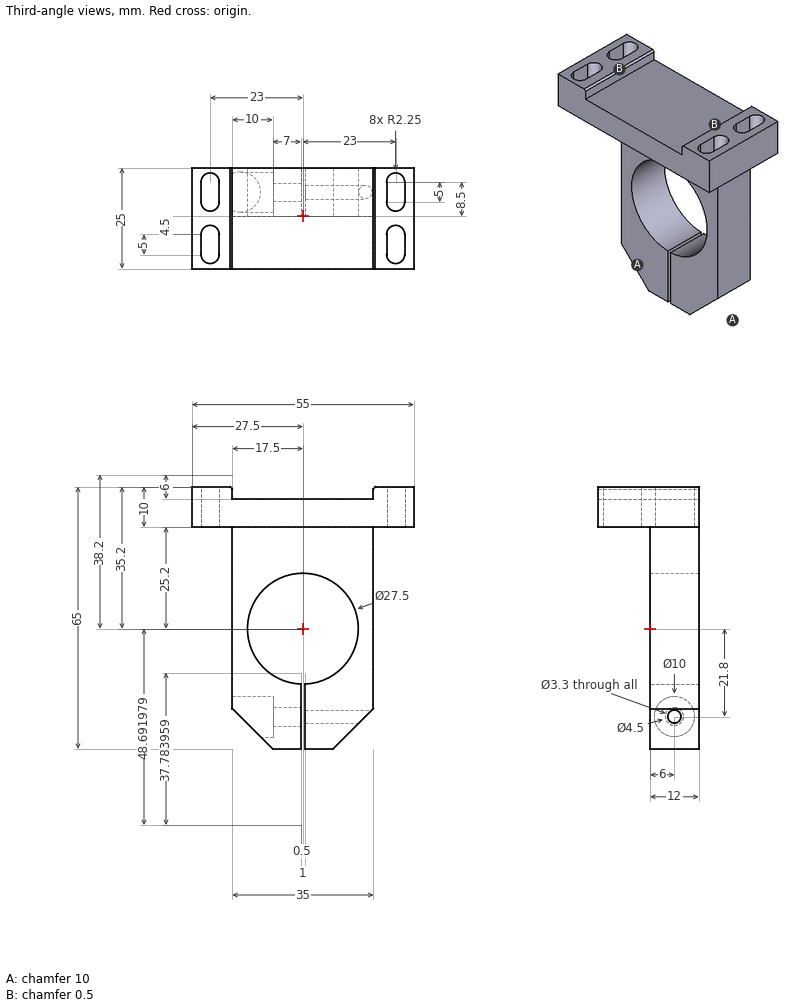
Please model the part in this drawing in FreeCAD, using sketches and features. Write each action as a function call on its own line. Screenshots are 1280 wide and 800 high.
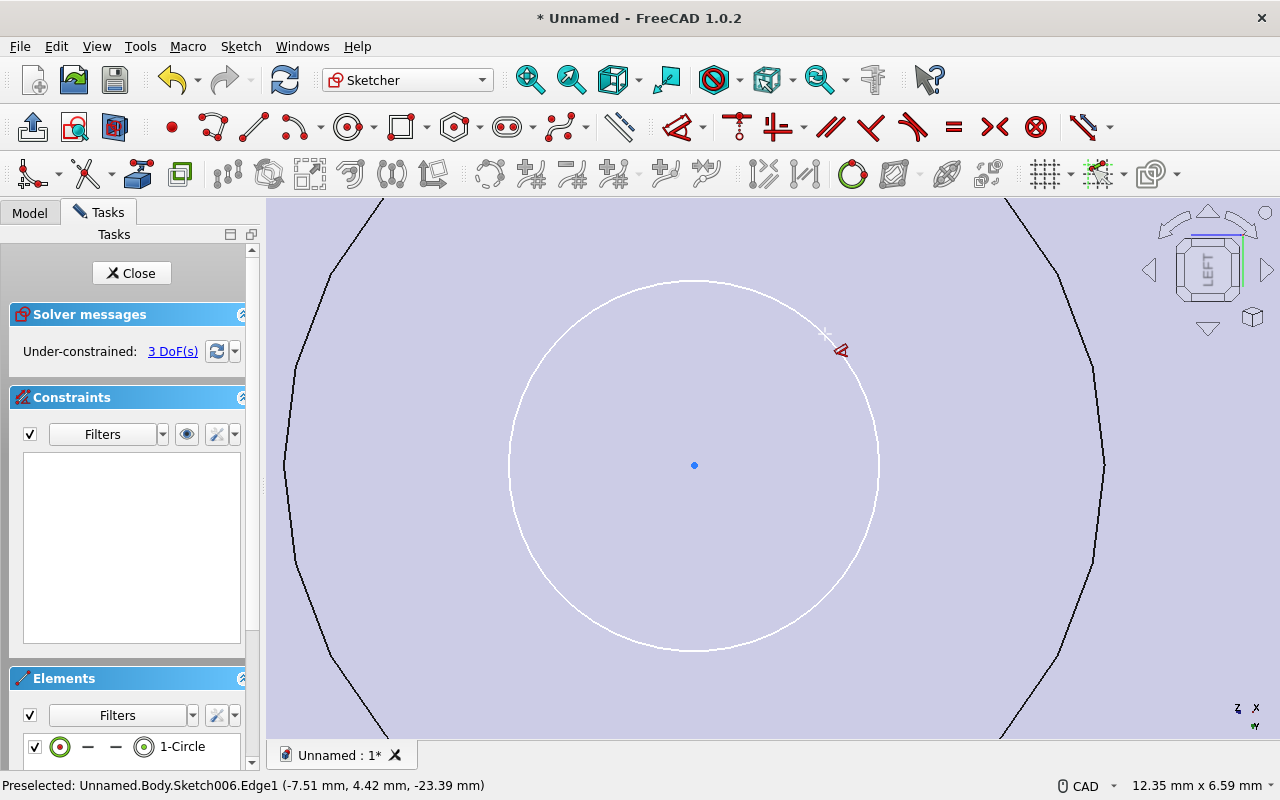
click(825, 335)
click(848, 312)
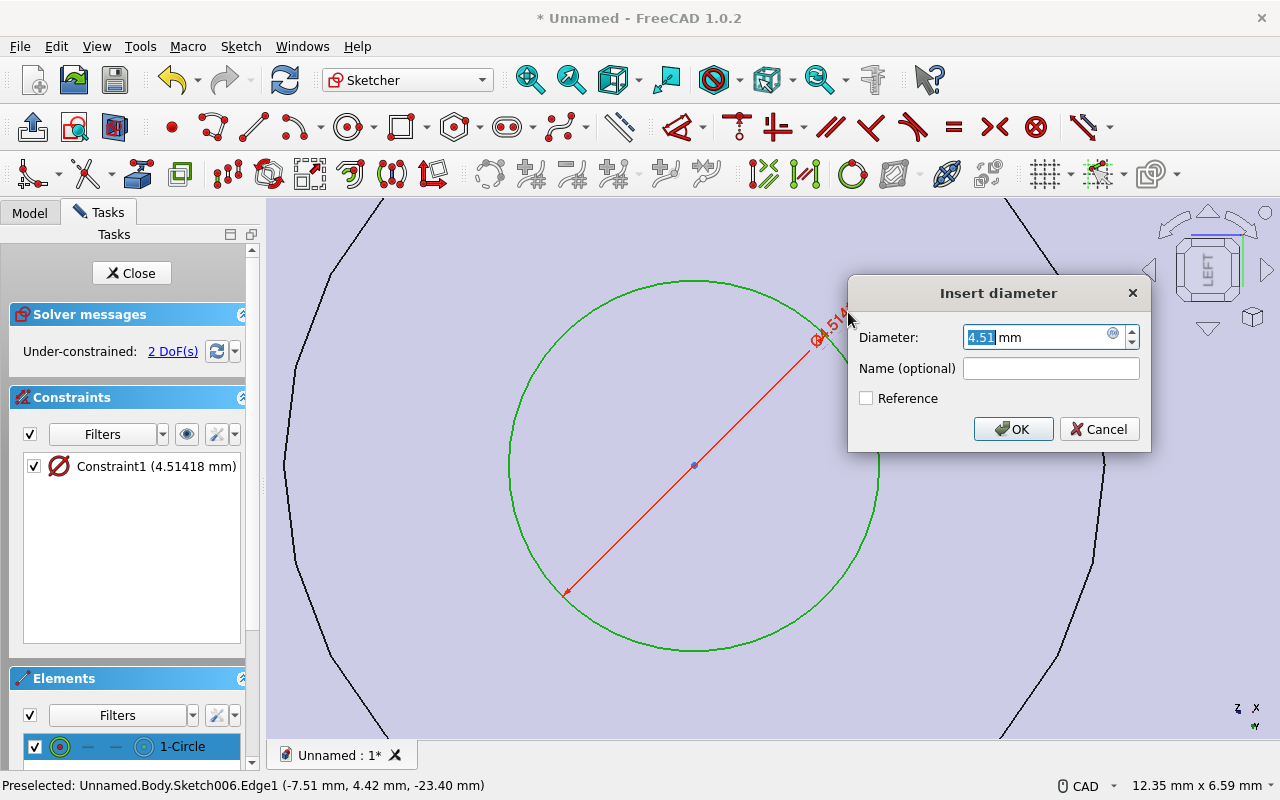
text(4.5)
key(Return)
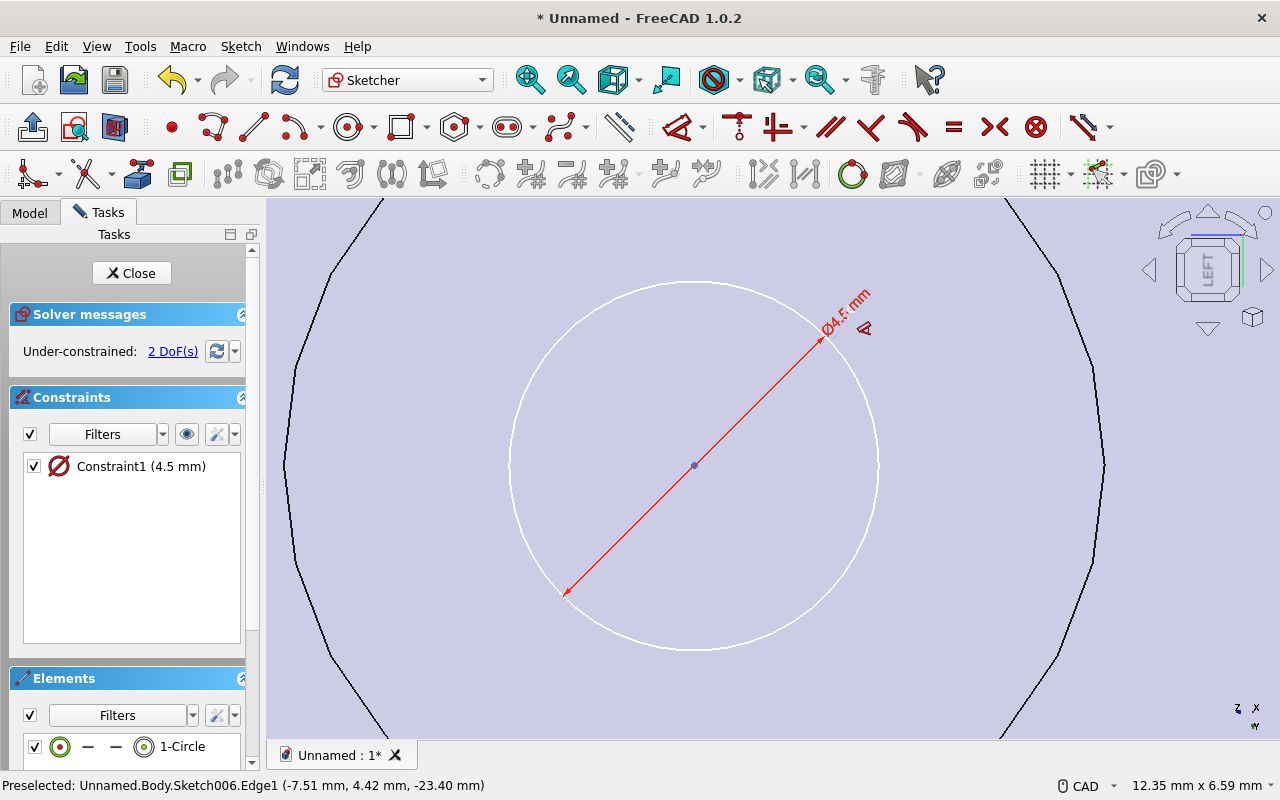
click(694, 466)
click(728, 346)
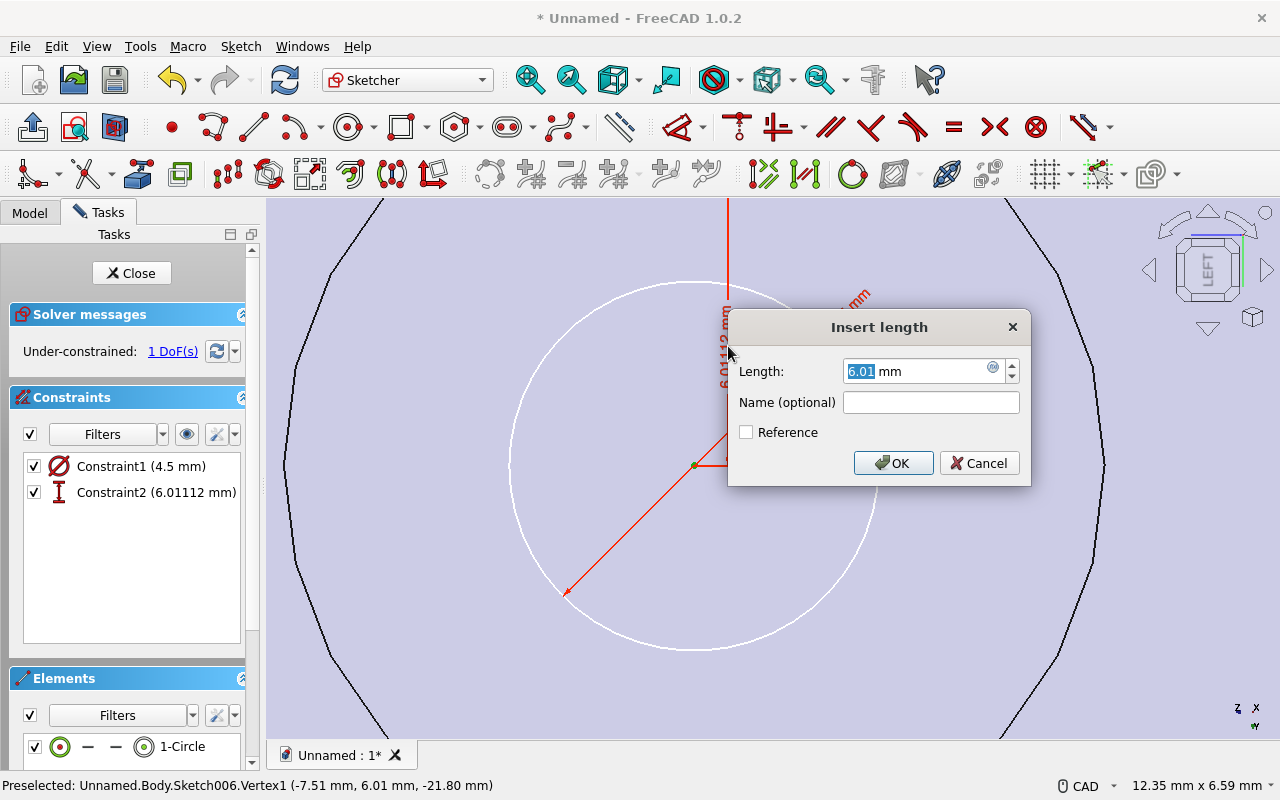
text(6)
key(Return)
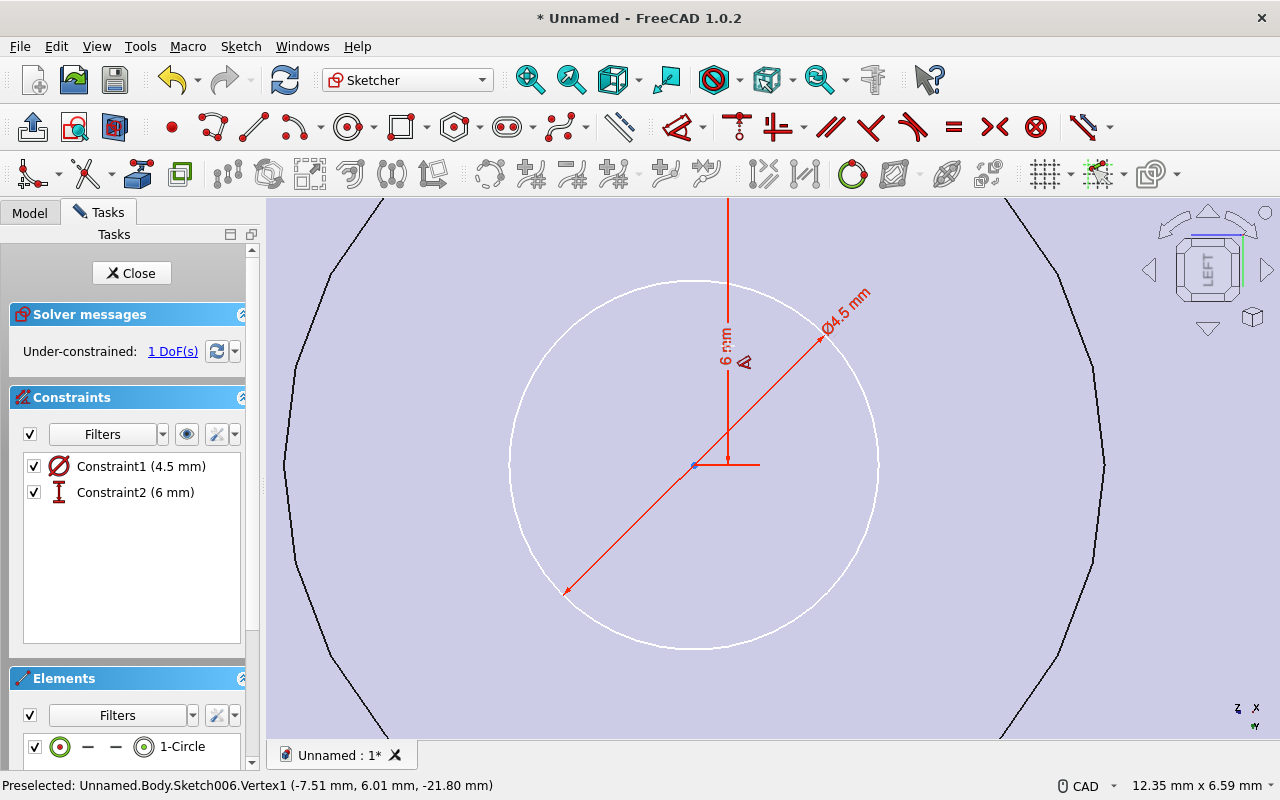
click(694, 465)
click(494, 499)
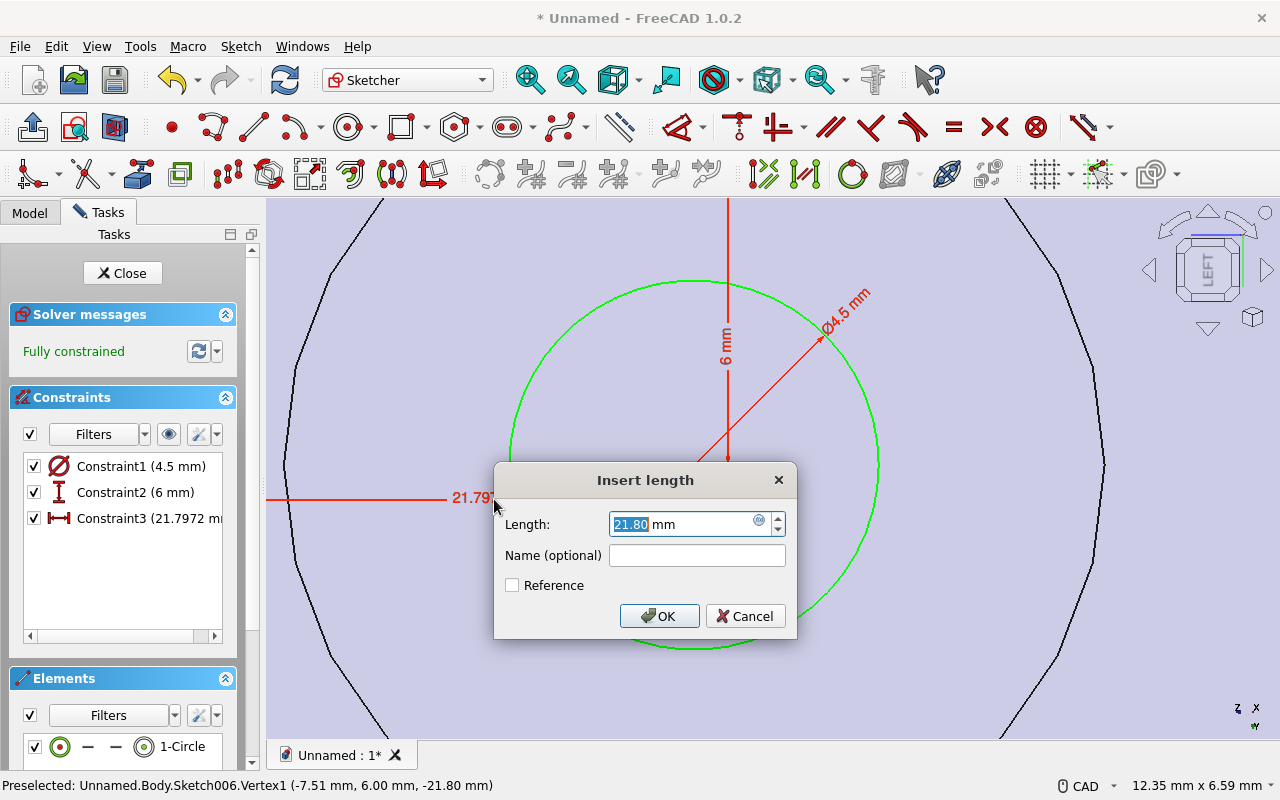
text(21.8)
key(Return)
key(Escape)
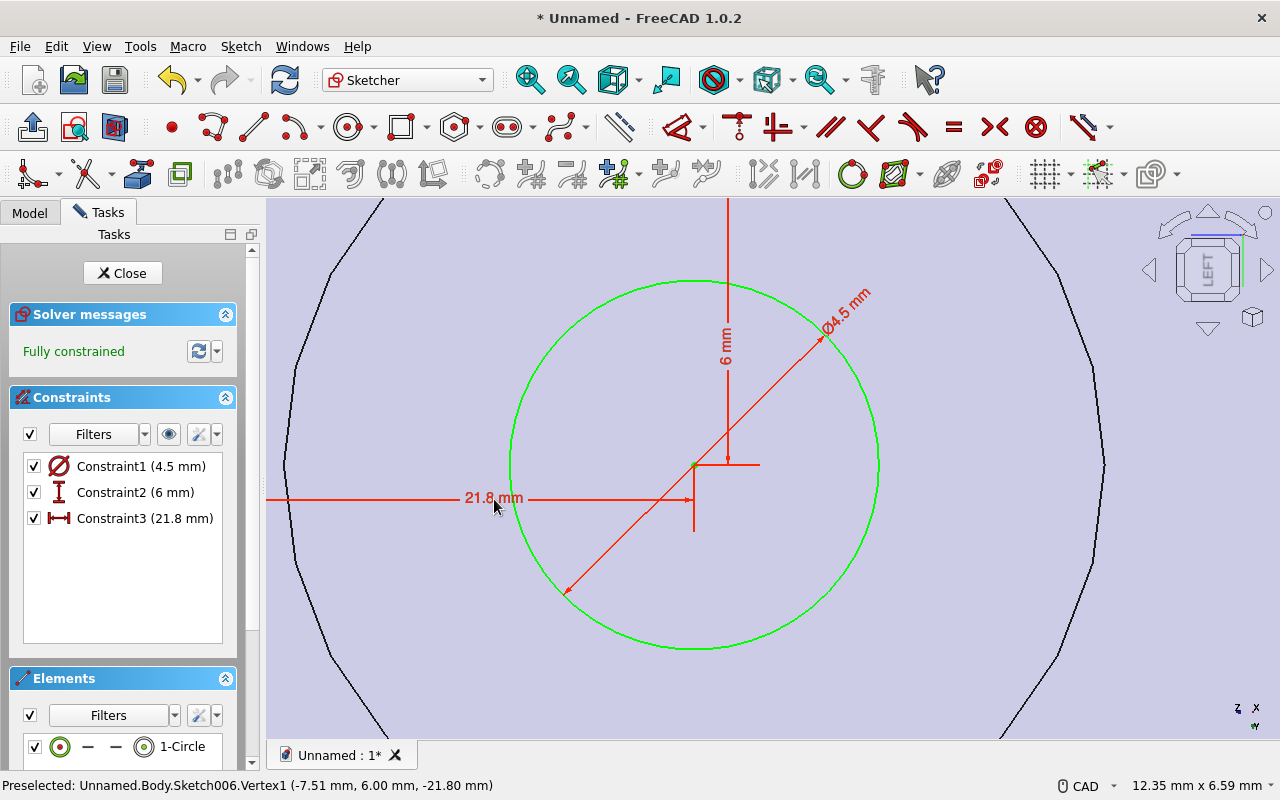
click(123, 273)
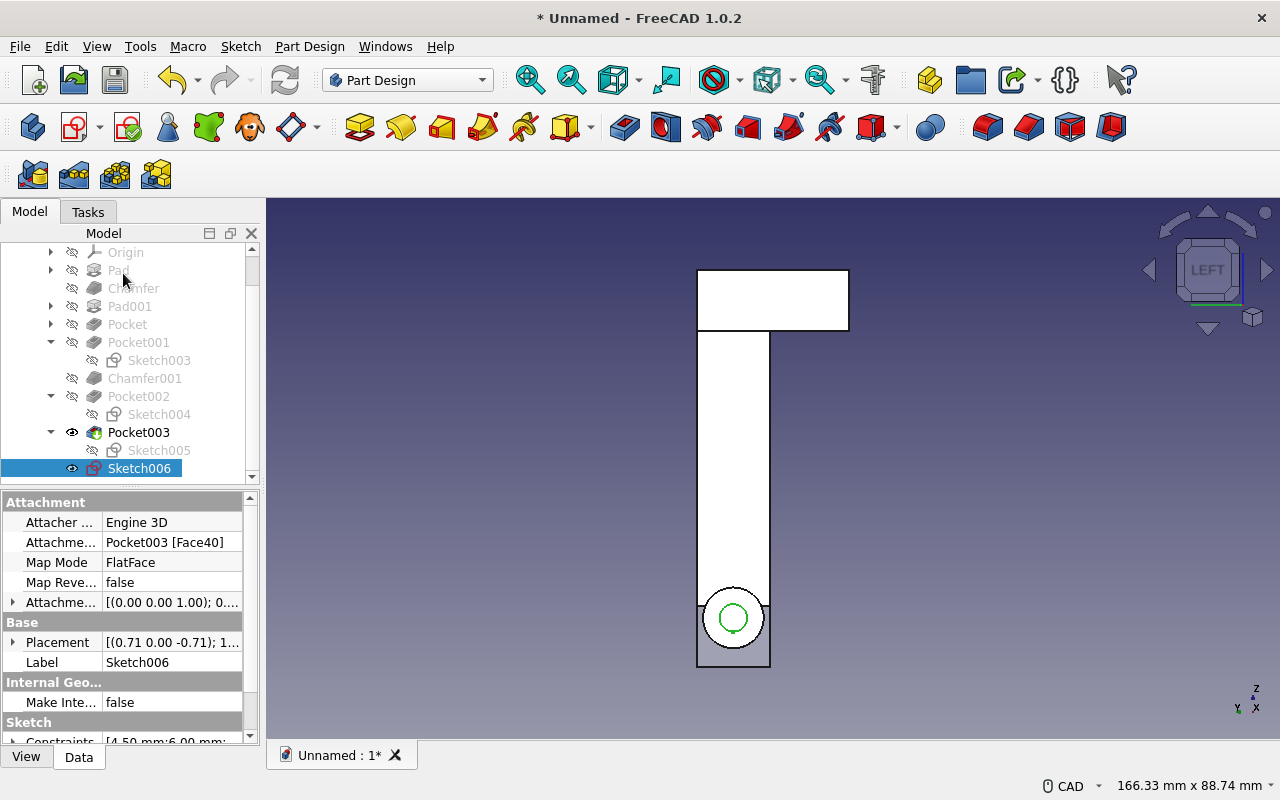
click(625, 128)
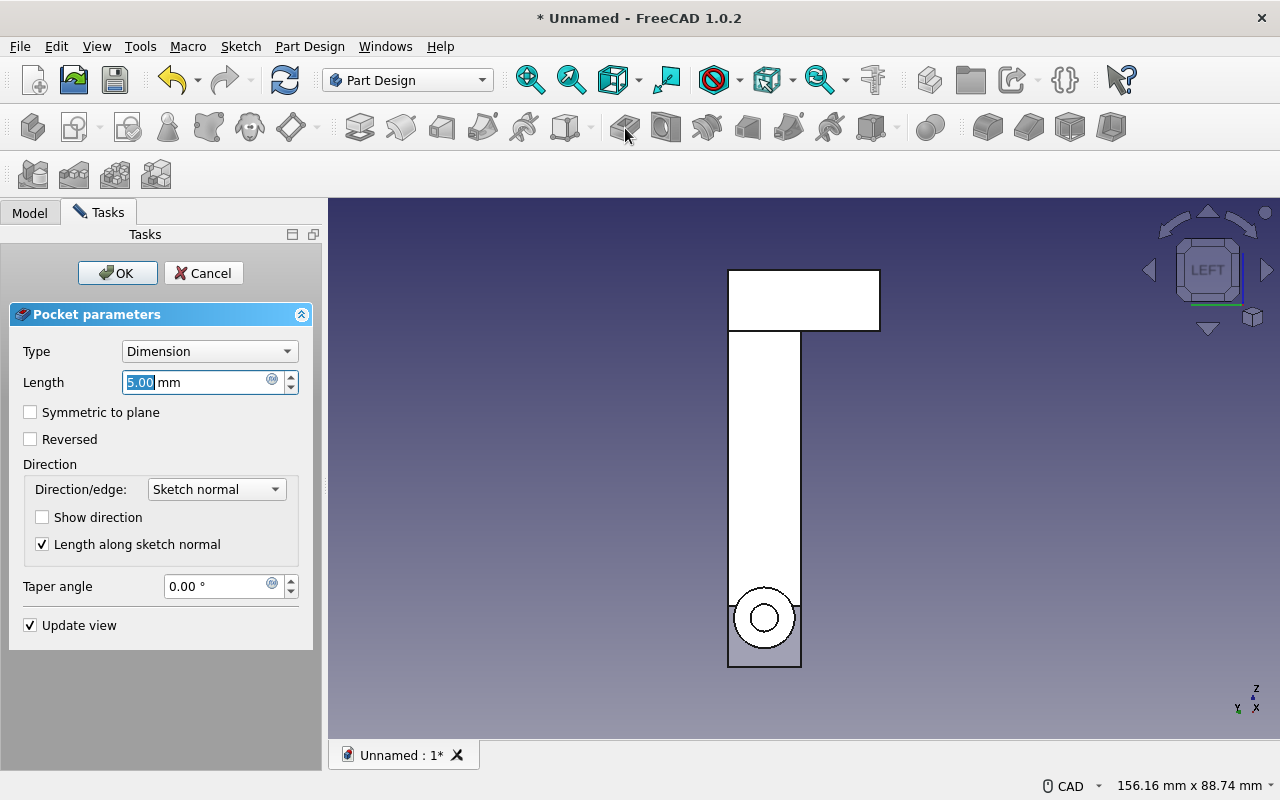
text(7)
key(Tab)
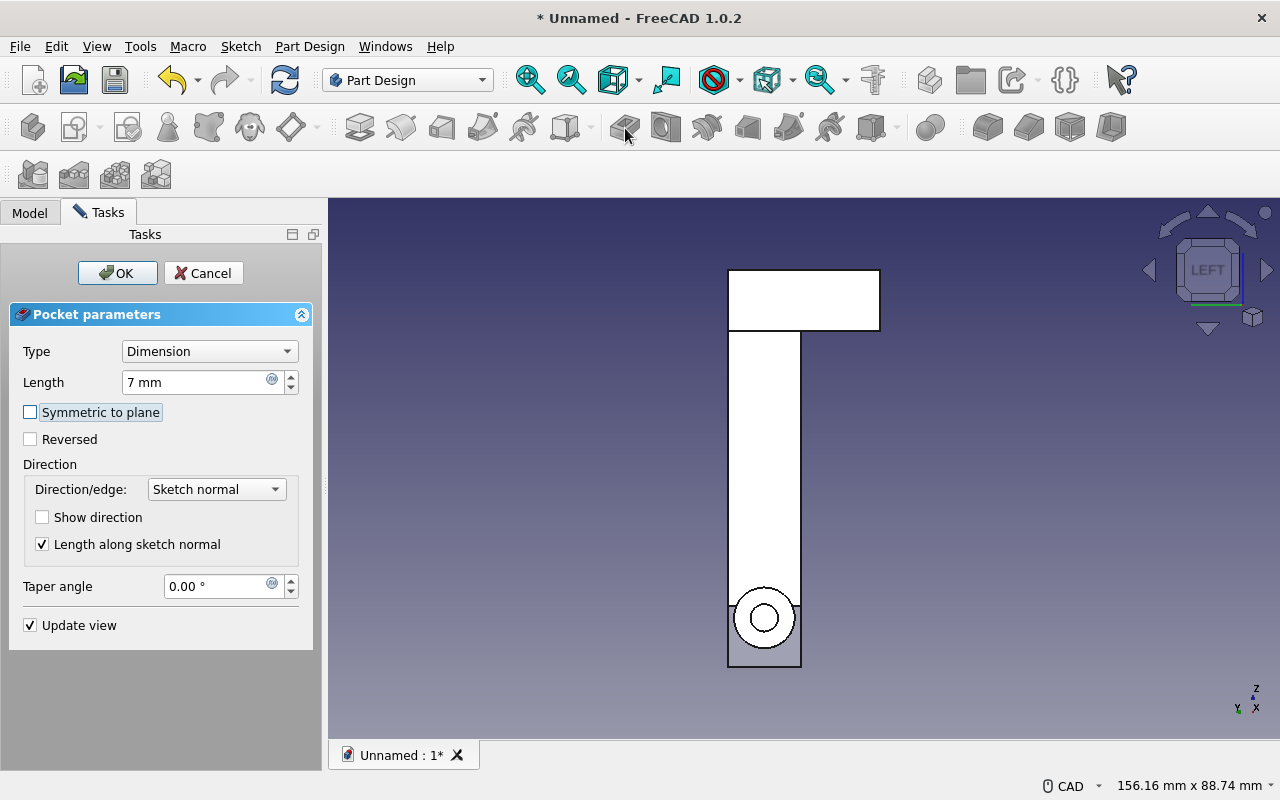
click(118, 273)